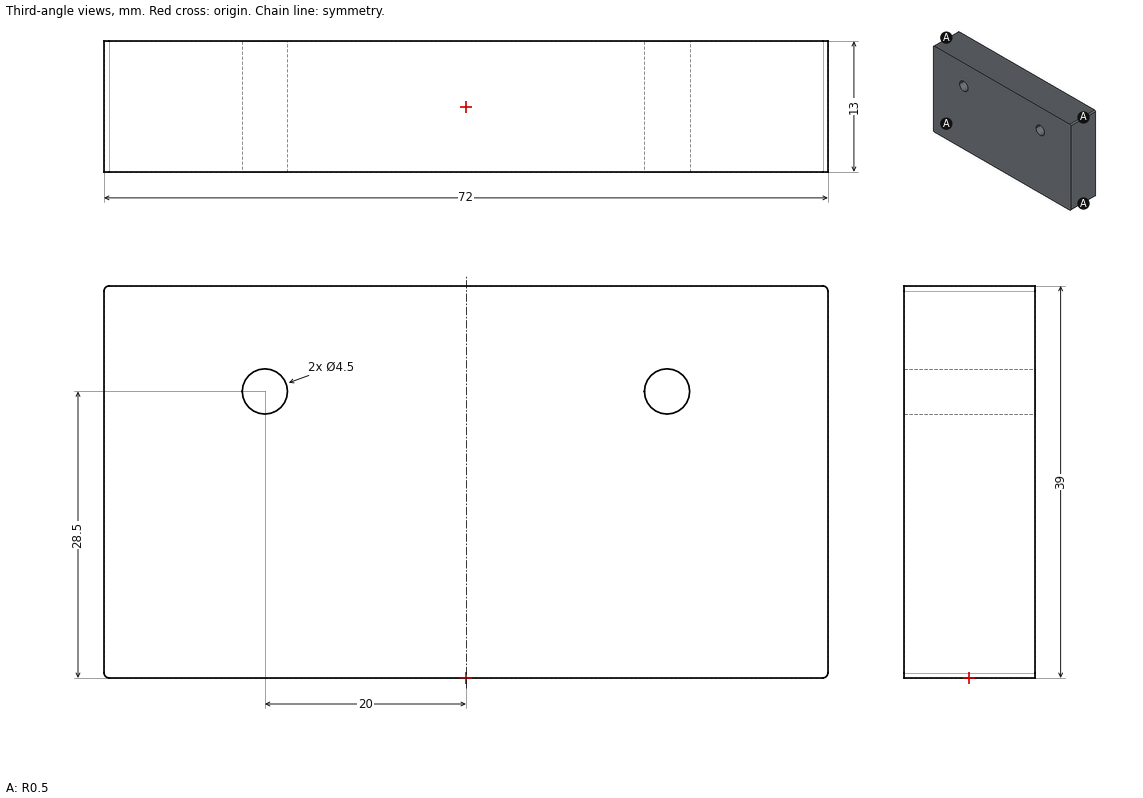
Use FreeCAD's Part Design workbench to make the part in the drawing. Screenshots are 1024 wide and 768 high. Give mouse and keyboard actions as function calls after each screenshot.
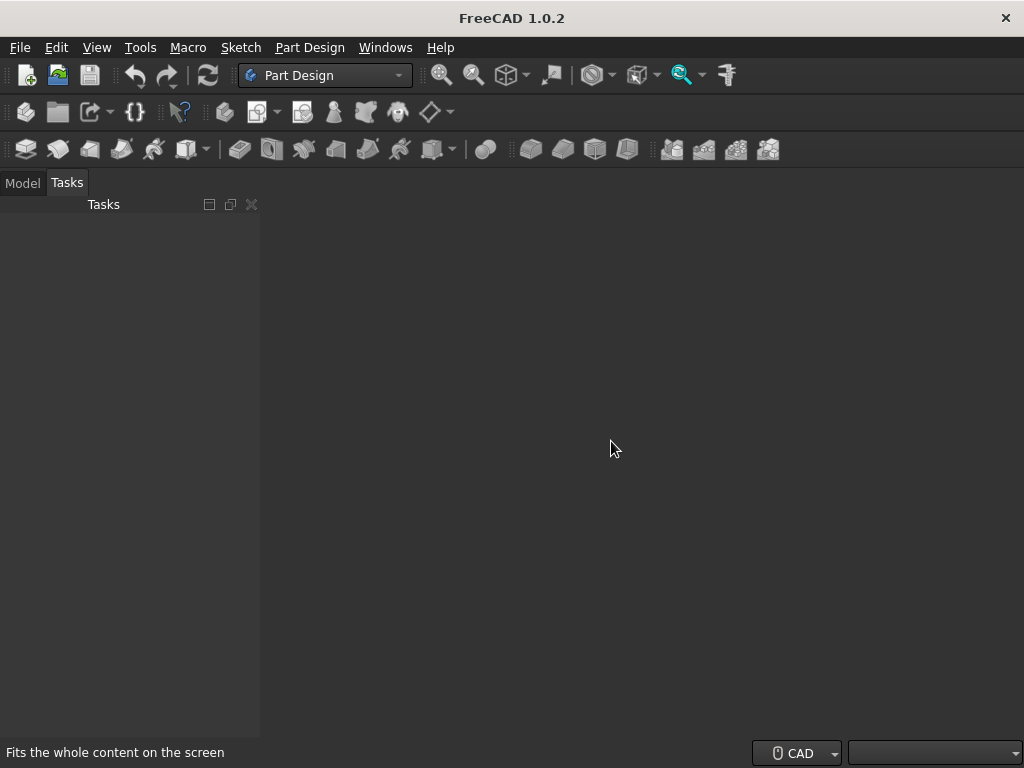
click(26, 76)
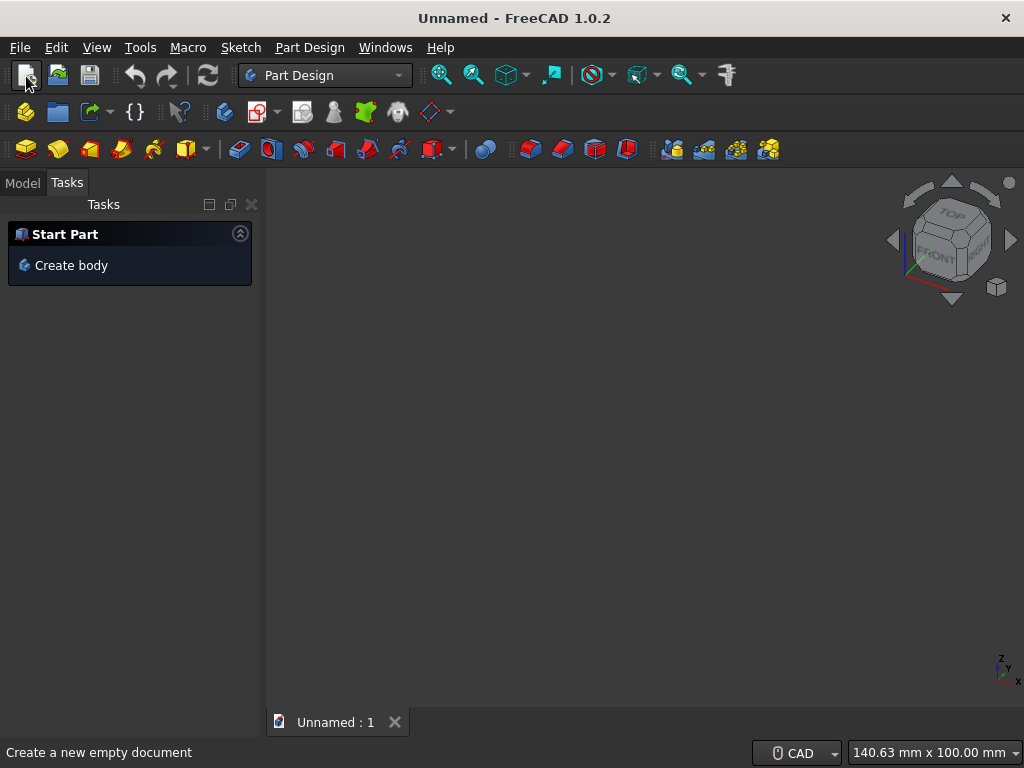
click(258, 112)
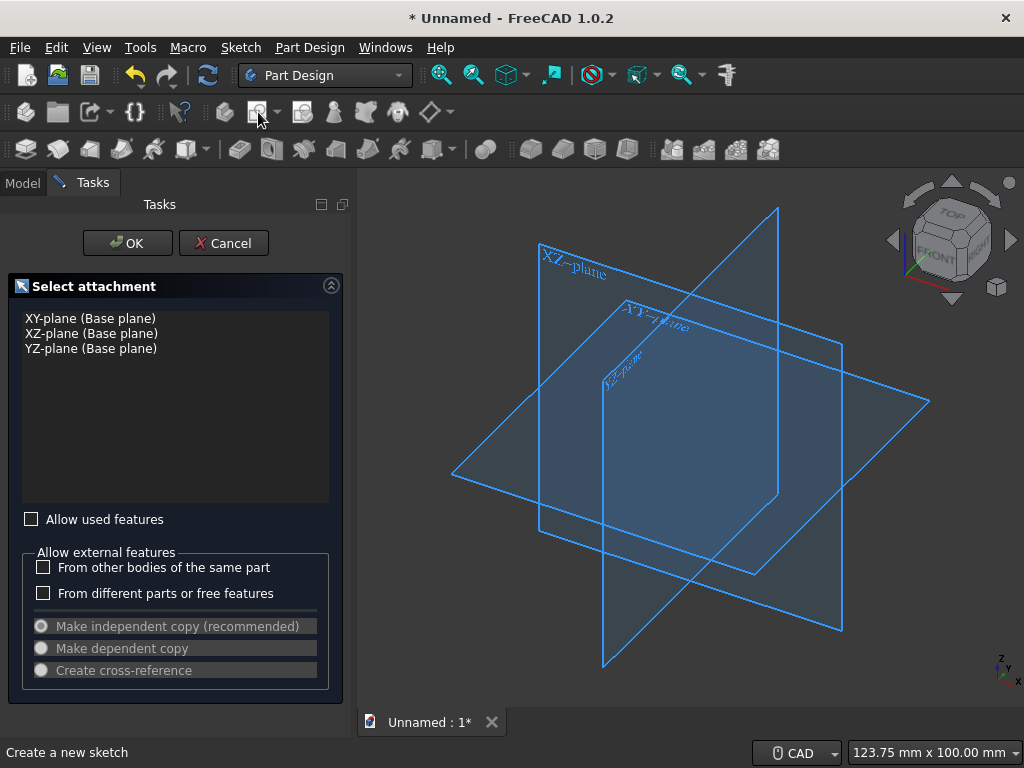
click(82, 318)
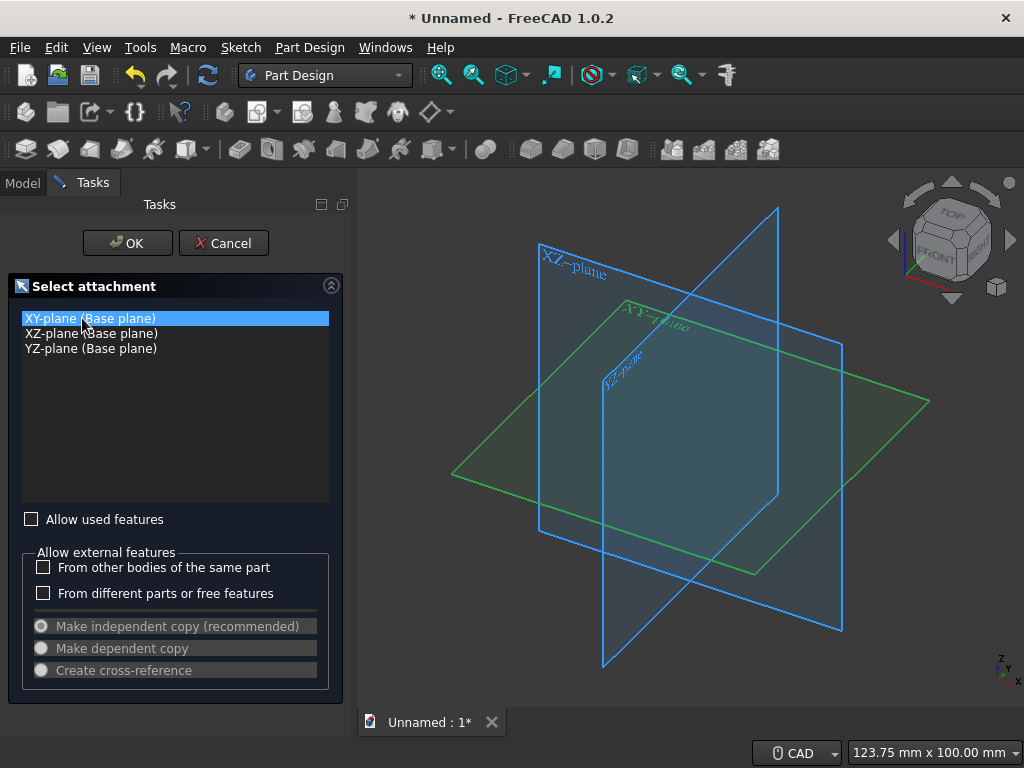
click(128, 243)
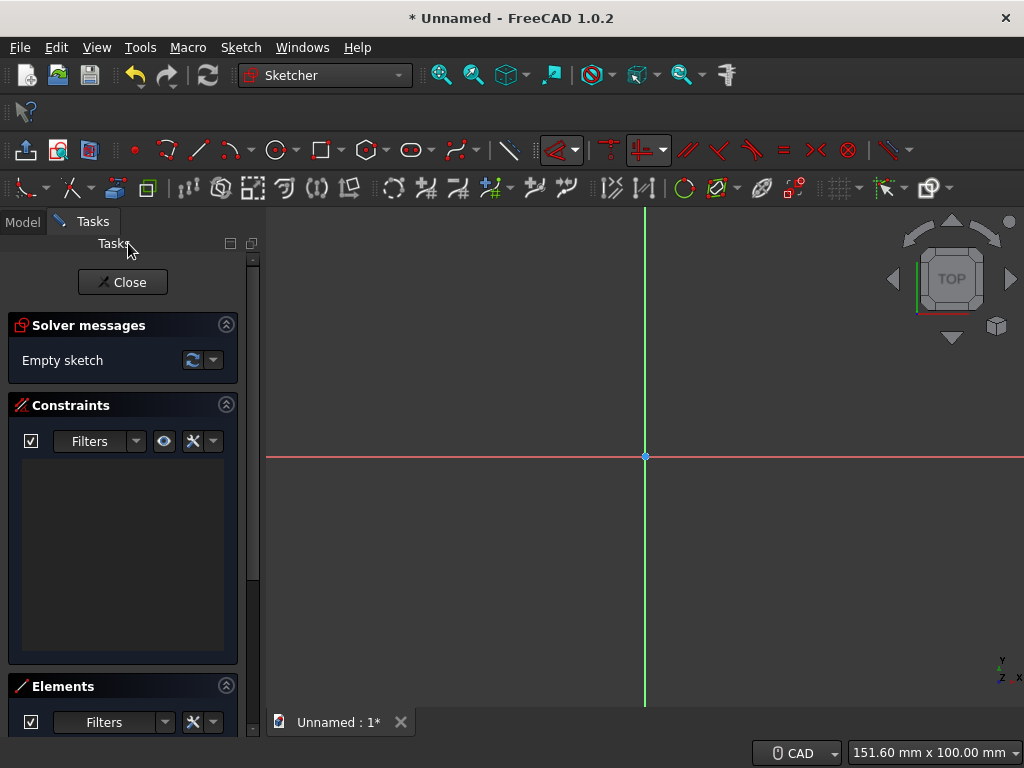
click(344, 150)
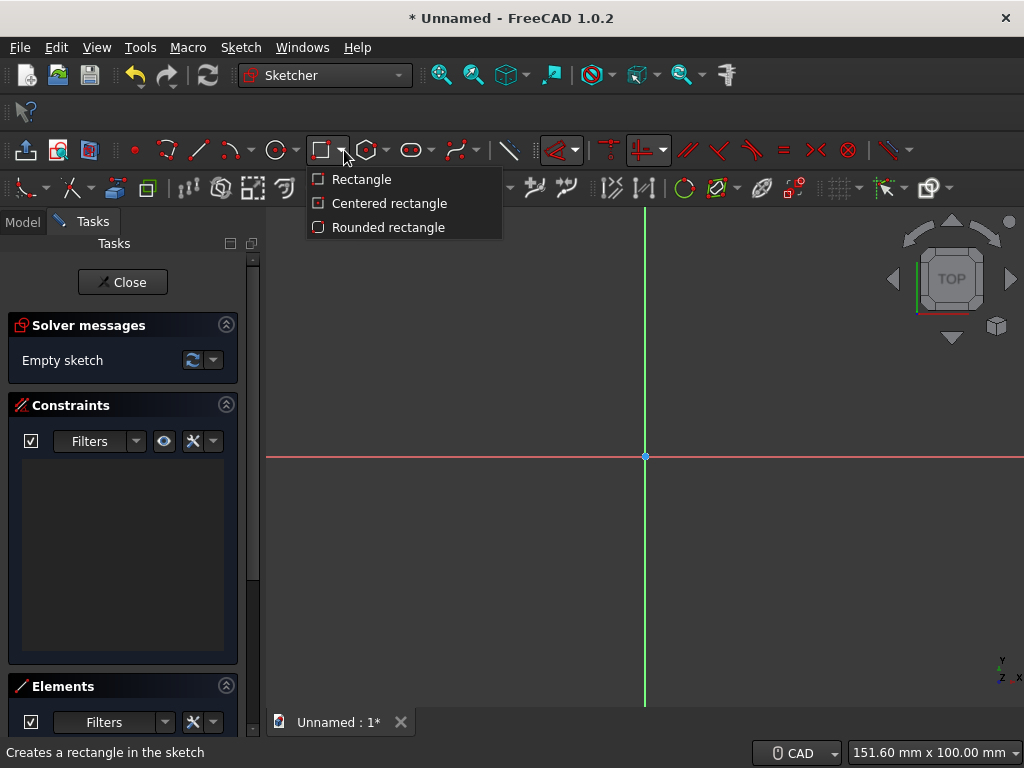
click(404, 203)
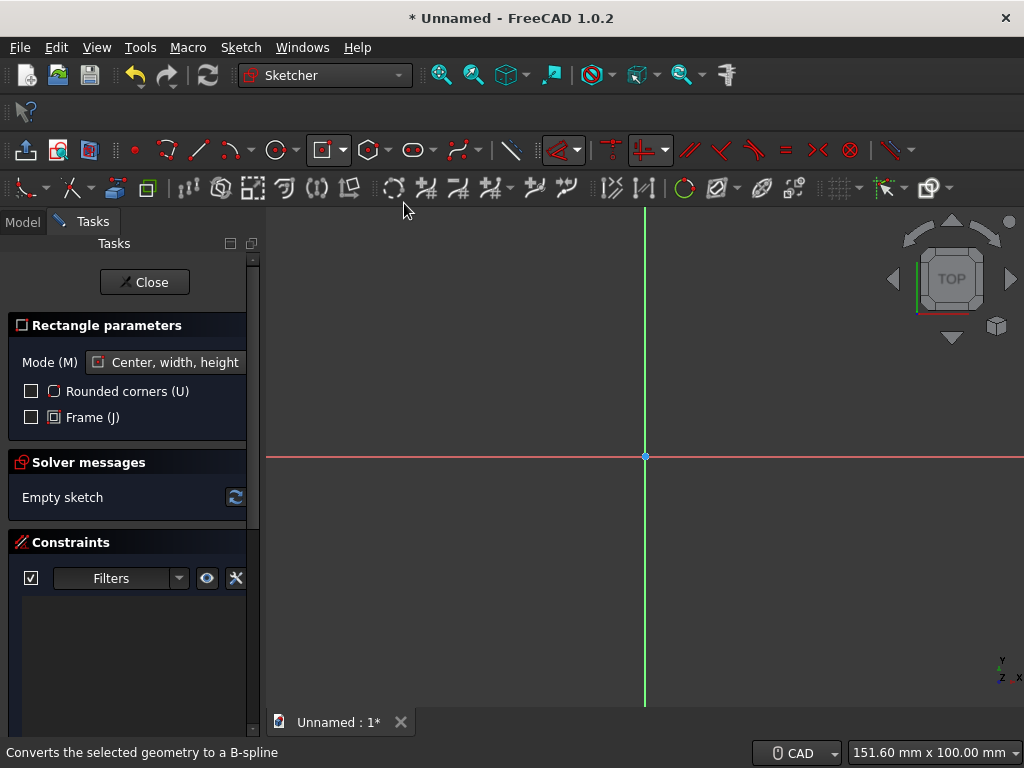
click(645, 457)
click(825, 424)
key(Escape)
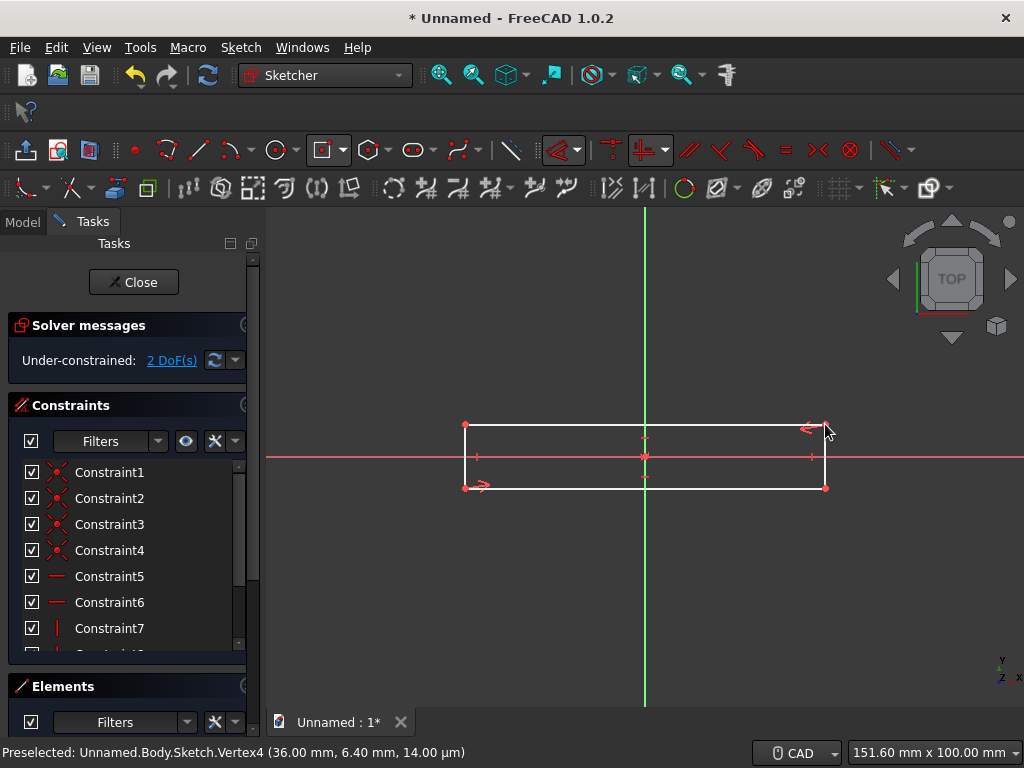
click(558, 150)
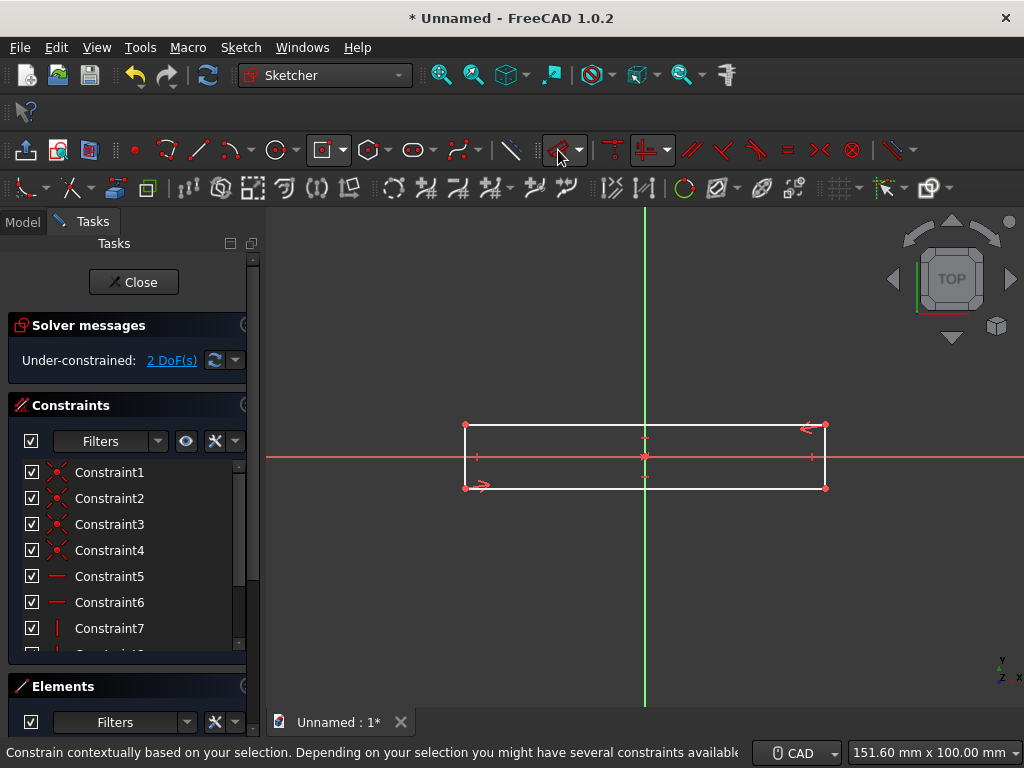
click(573, 489)
click(562, 523)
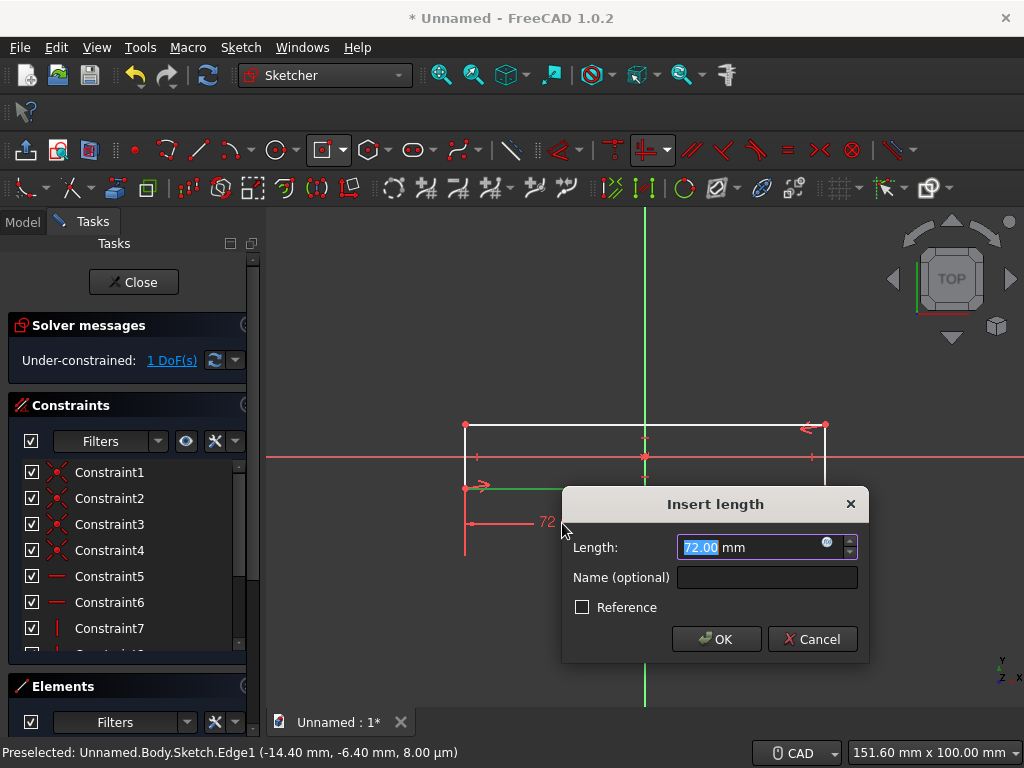
text(72)
key(Return)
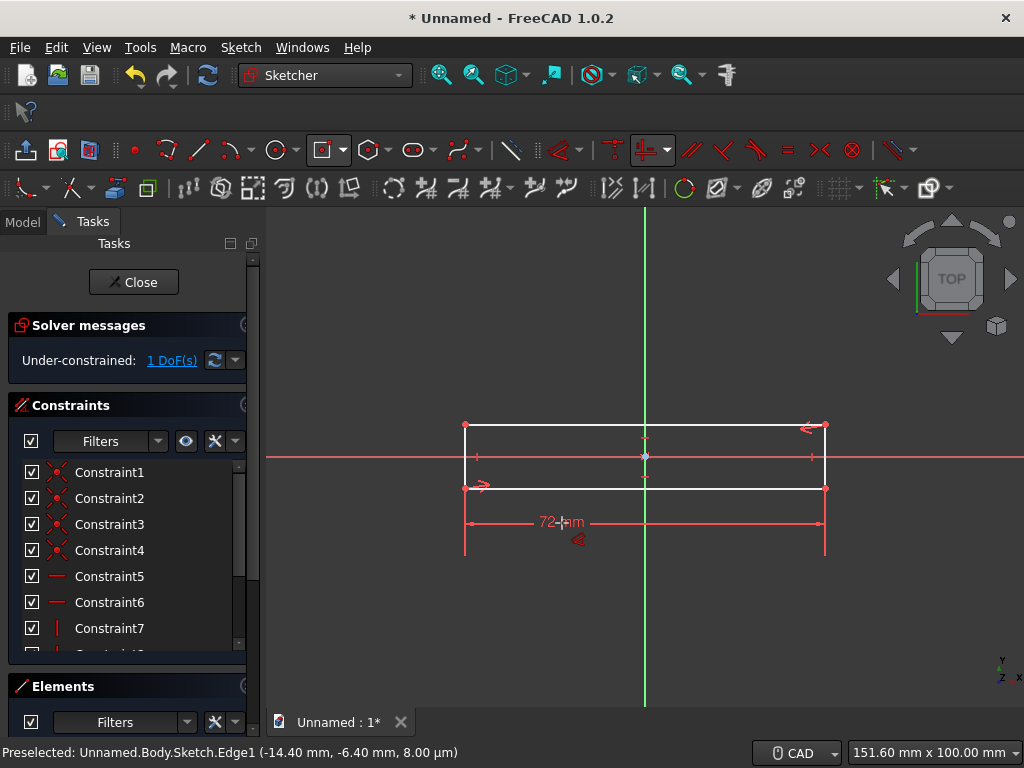
click(825, 470)
click(859, 442)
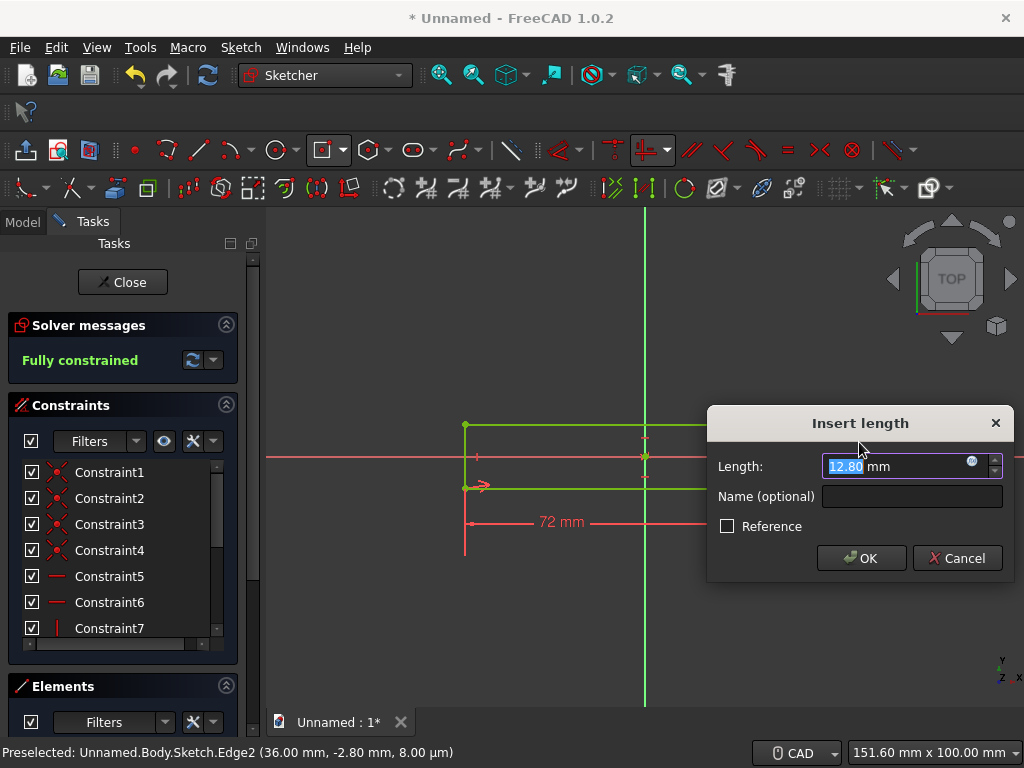
text(13)
key(Return)
key(Escape)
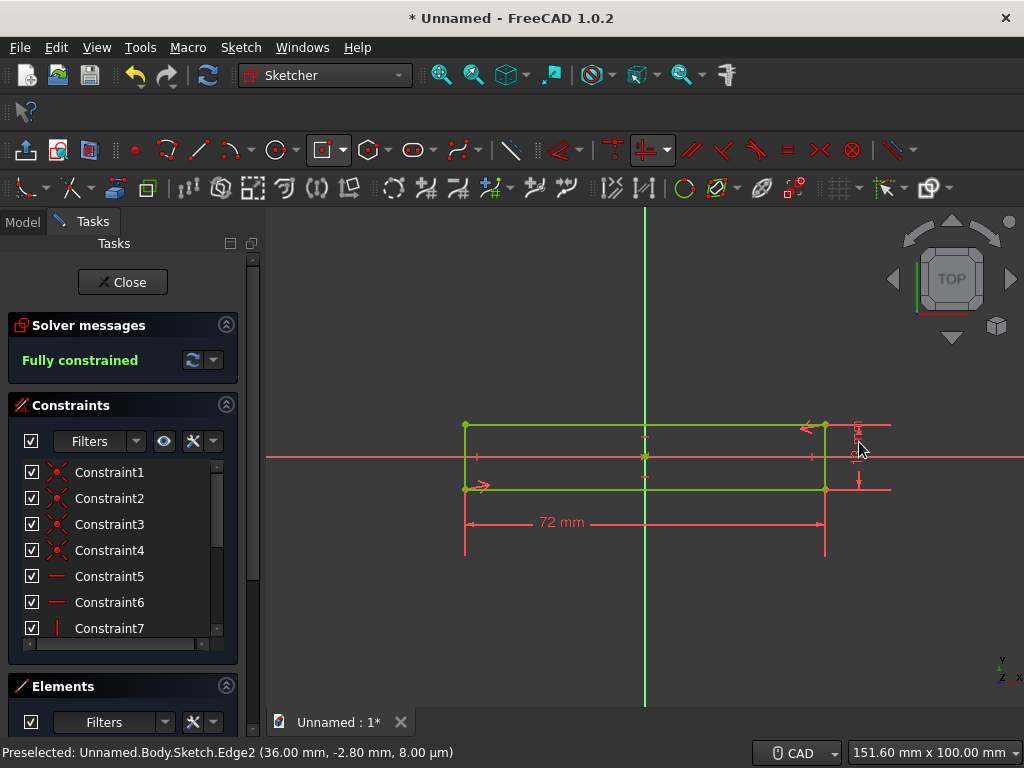
click(123, 282)